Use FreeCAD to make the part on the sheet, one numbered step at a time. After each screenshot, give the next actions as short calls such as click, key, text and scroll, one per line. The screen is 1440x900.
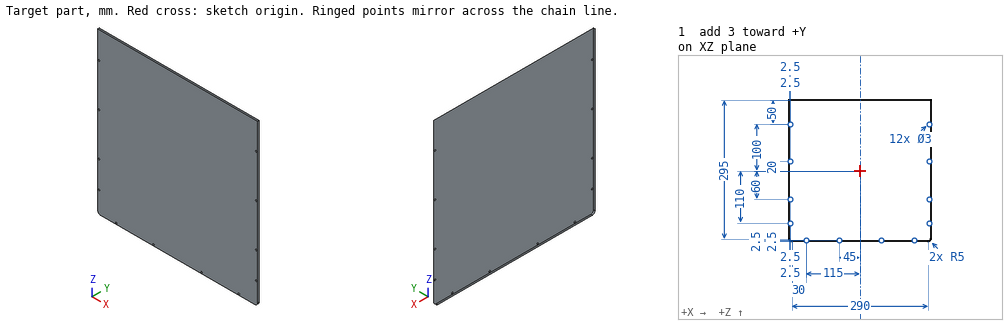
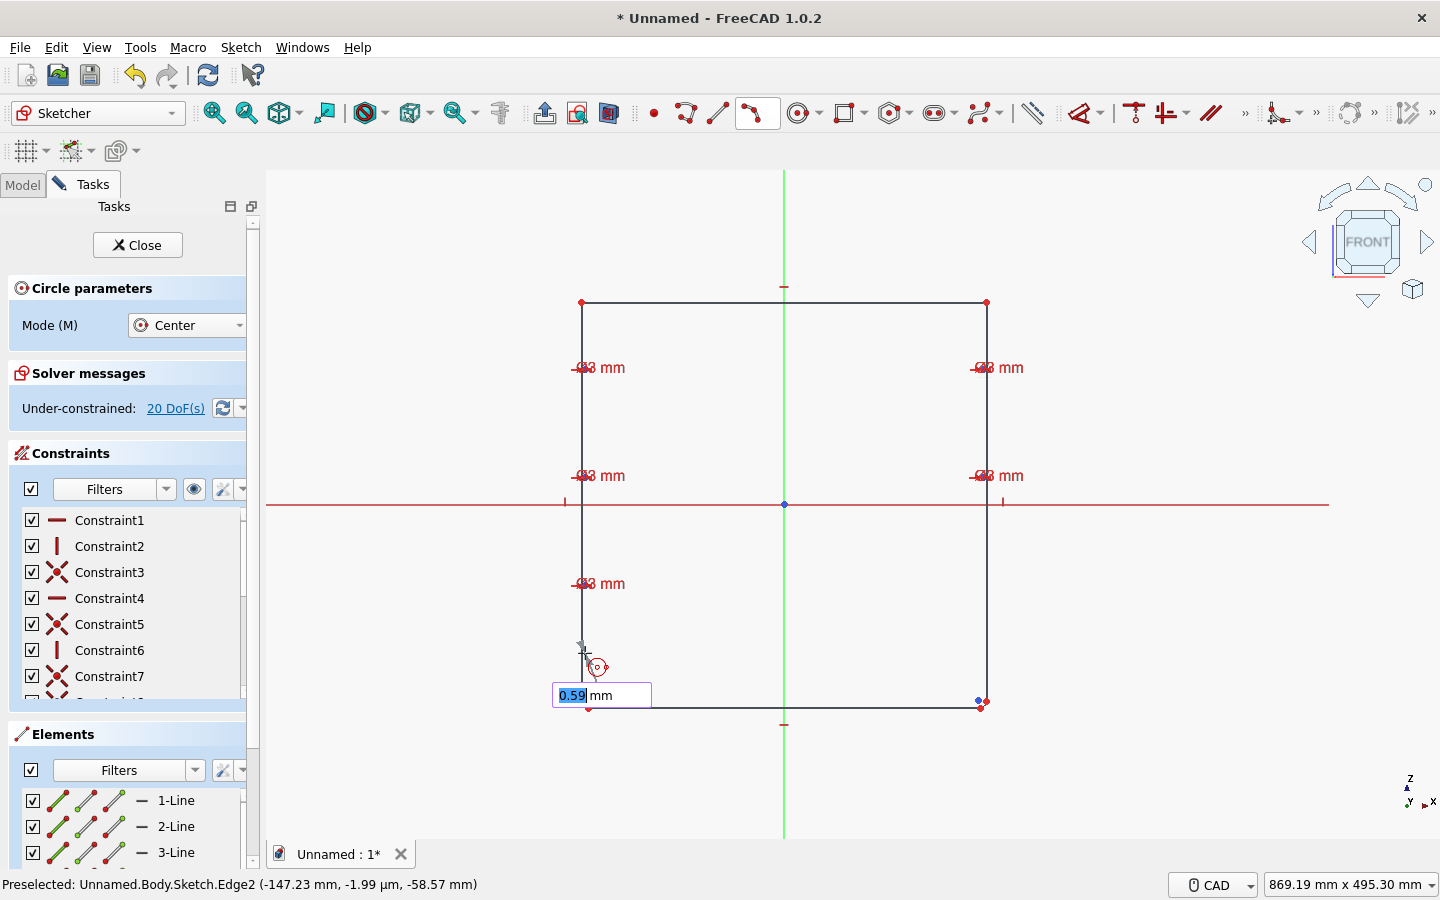
scroll(587, 652, up, 6)
move(585, 650)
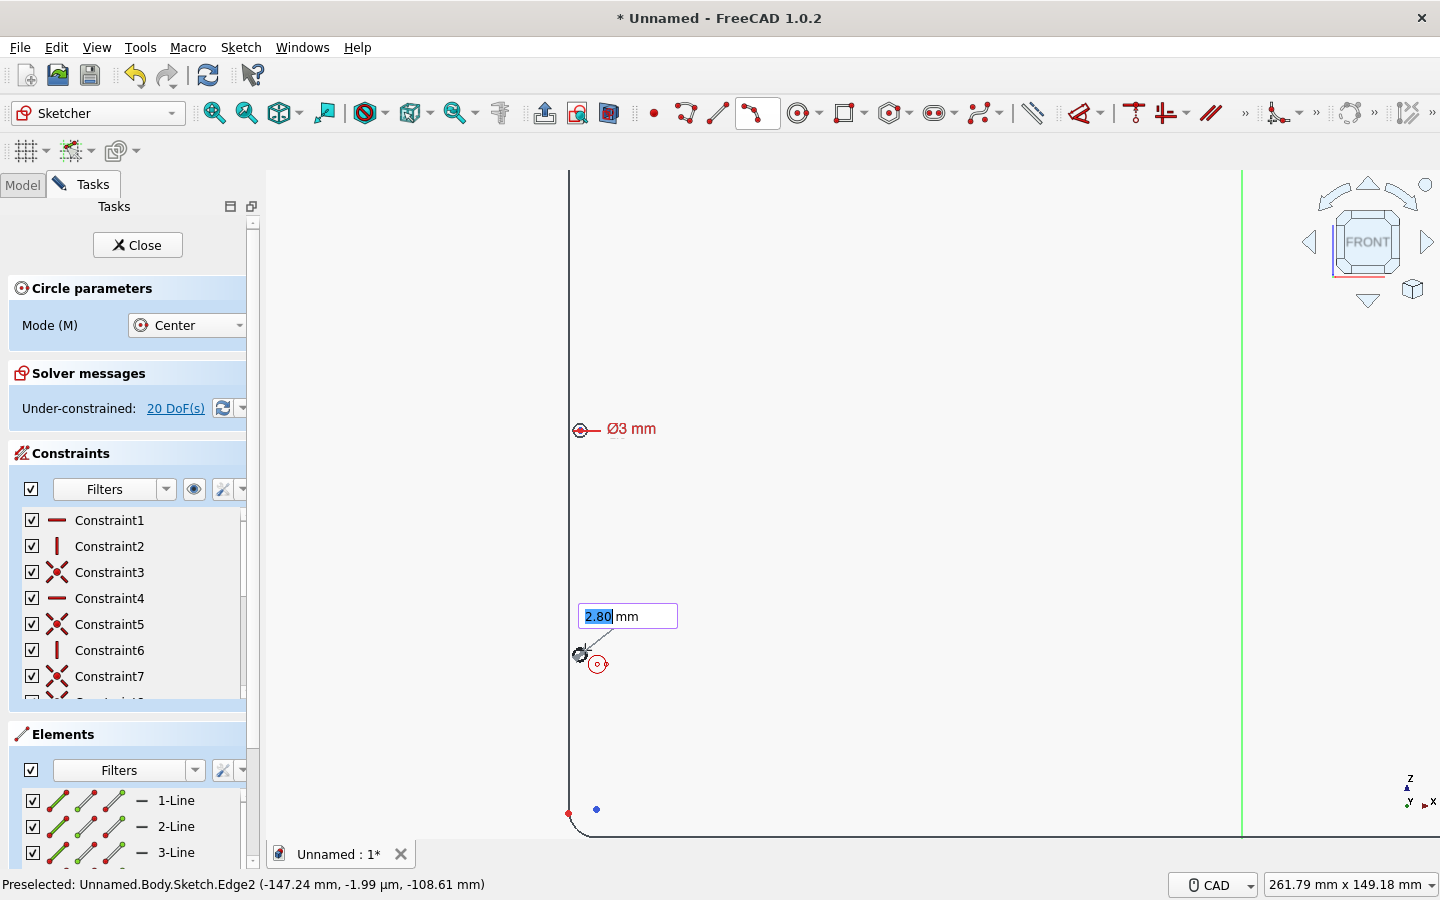
text(3)
key(Return)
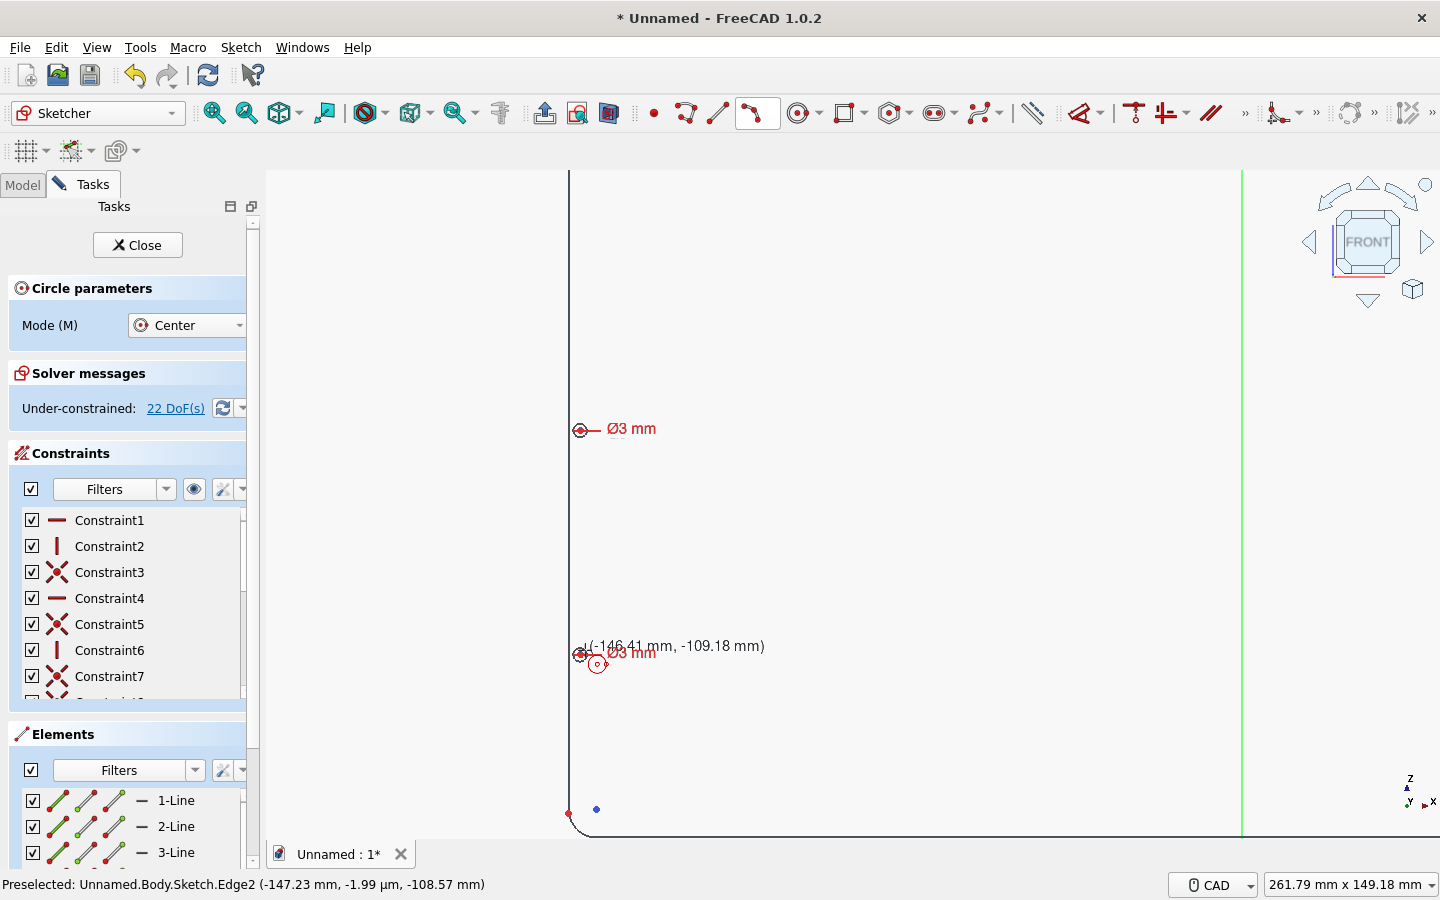
scroll(587, 652, down, 6)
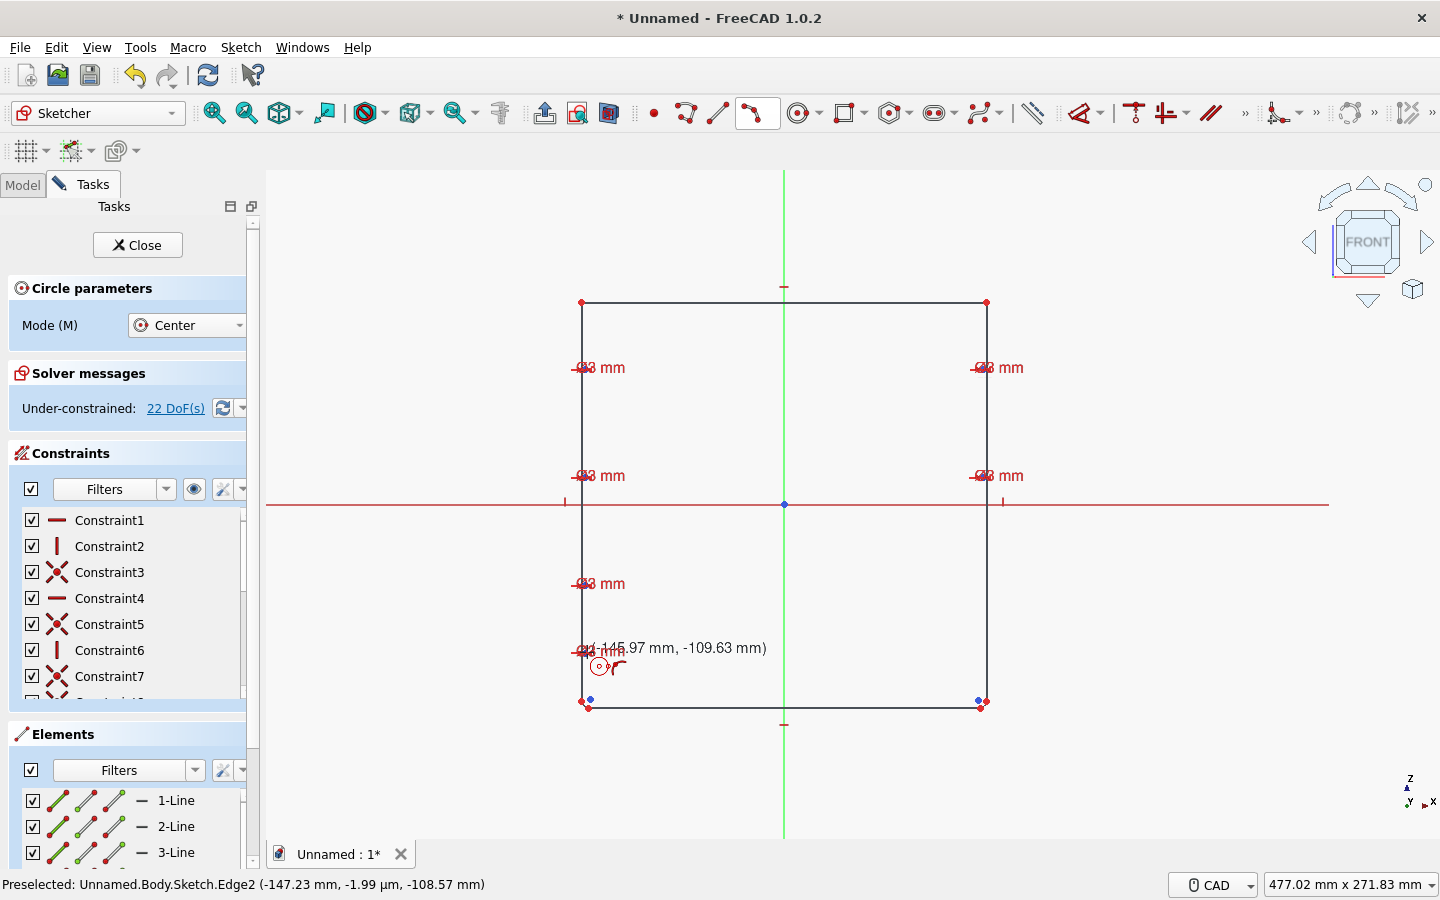
scroll(629, 704, up, 13)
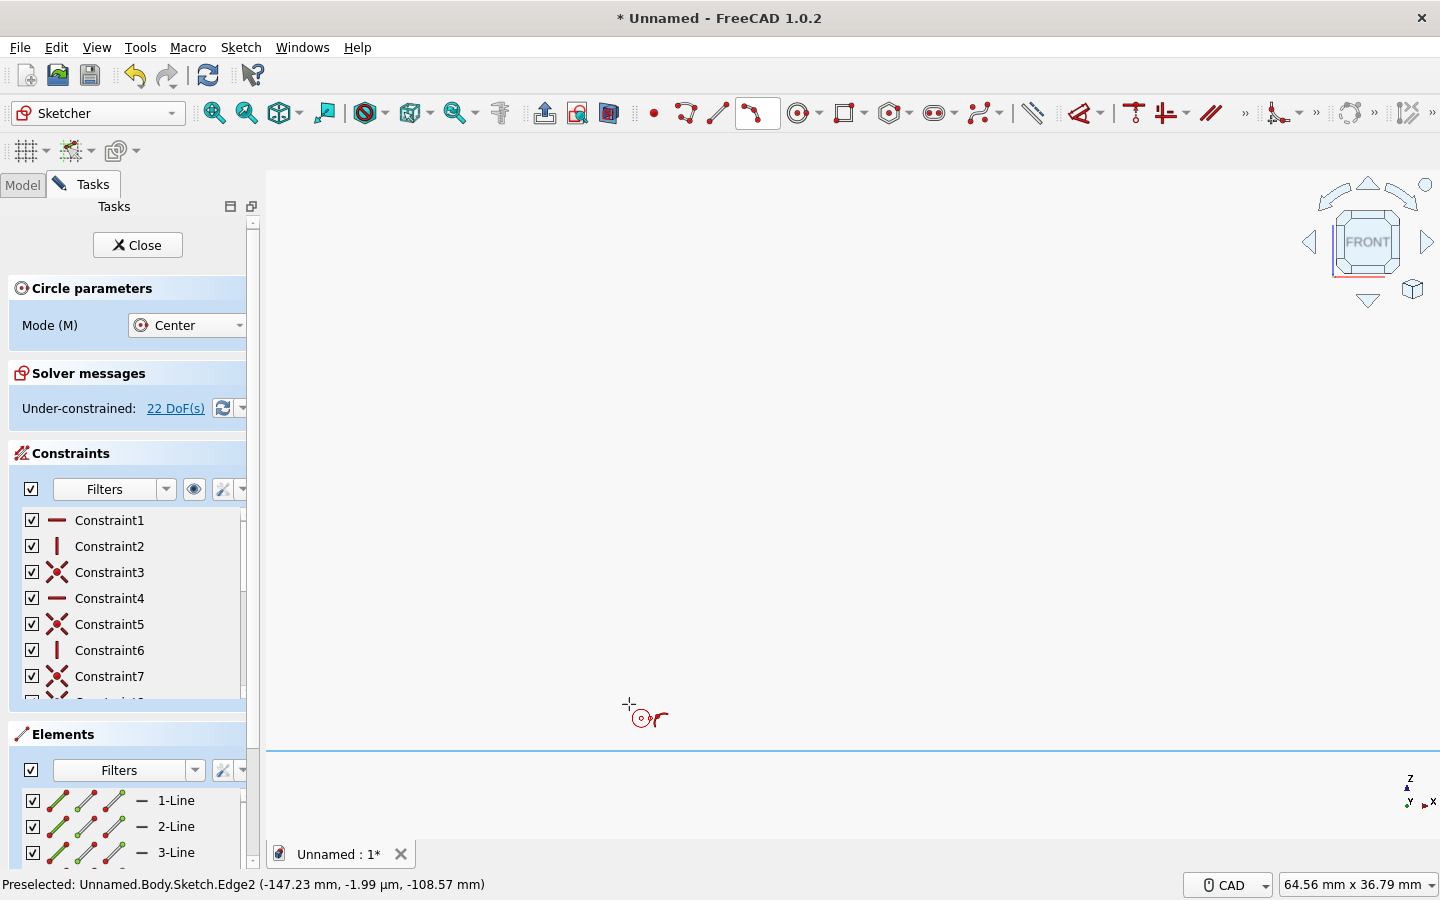
click(625, 694)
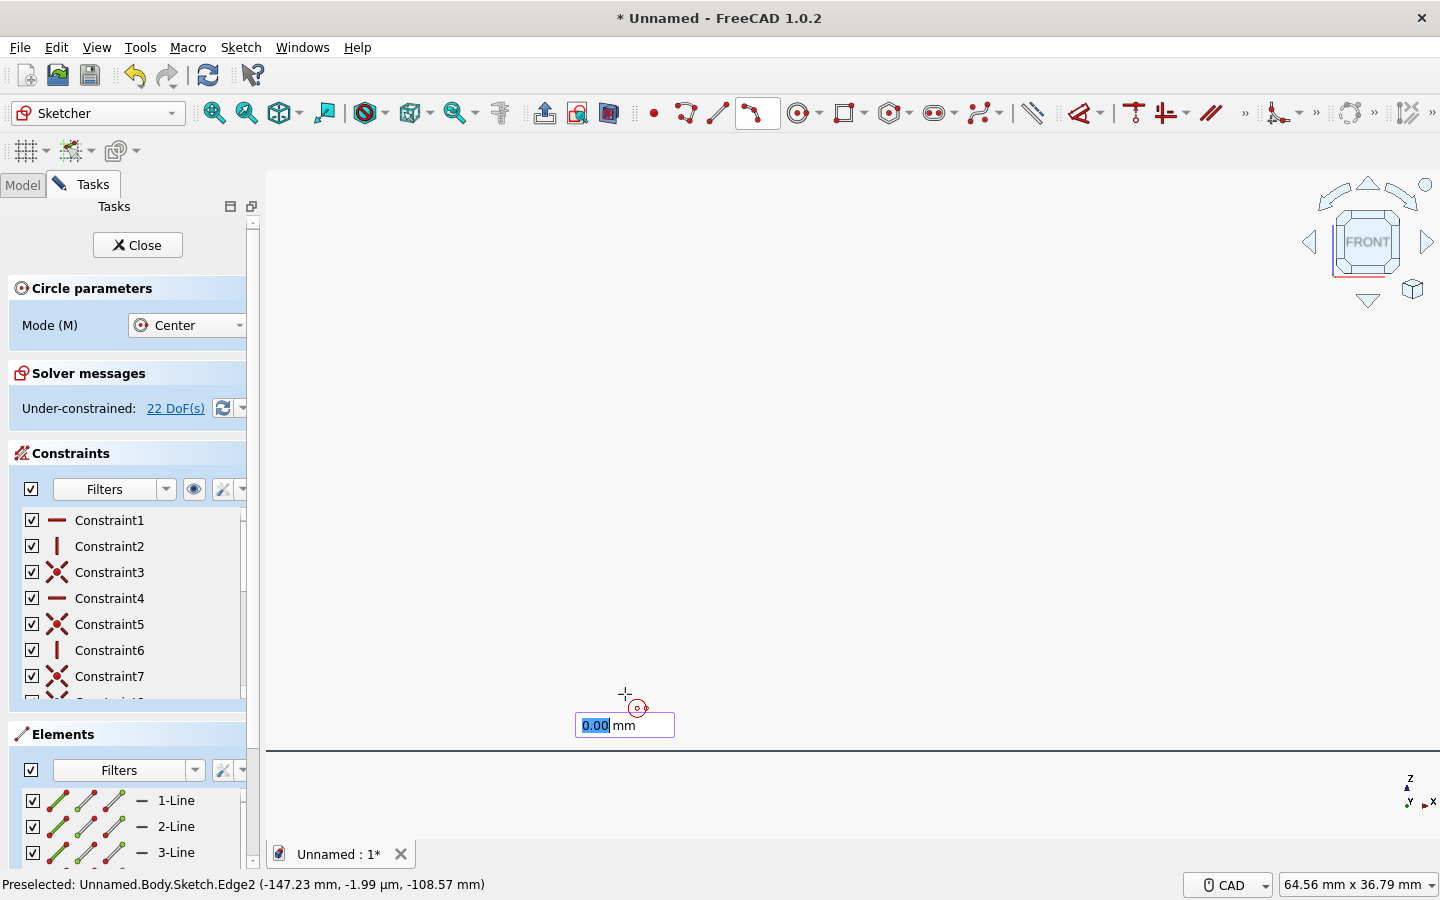
scroll(629, 705, down, 13)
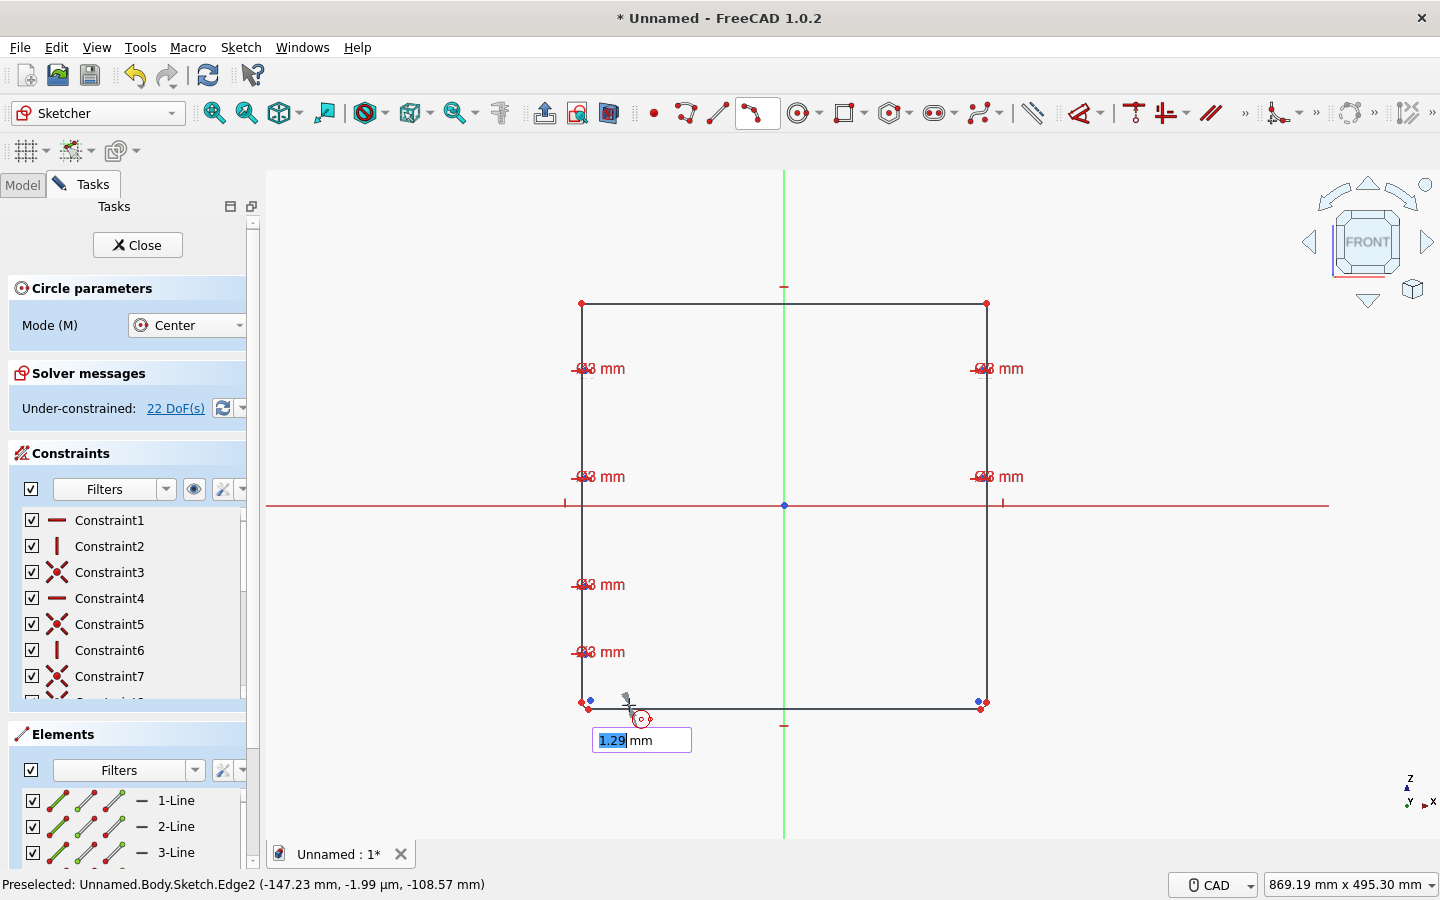
scroll(630, 703, up, 6)
move(631, 703)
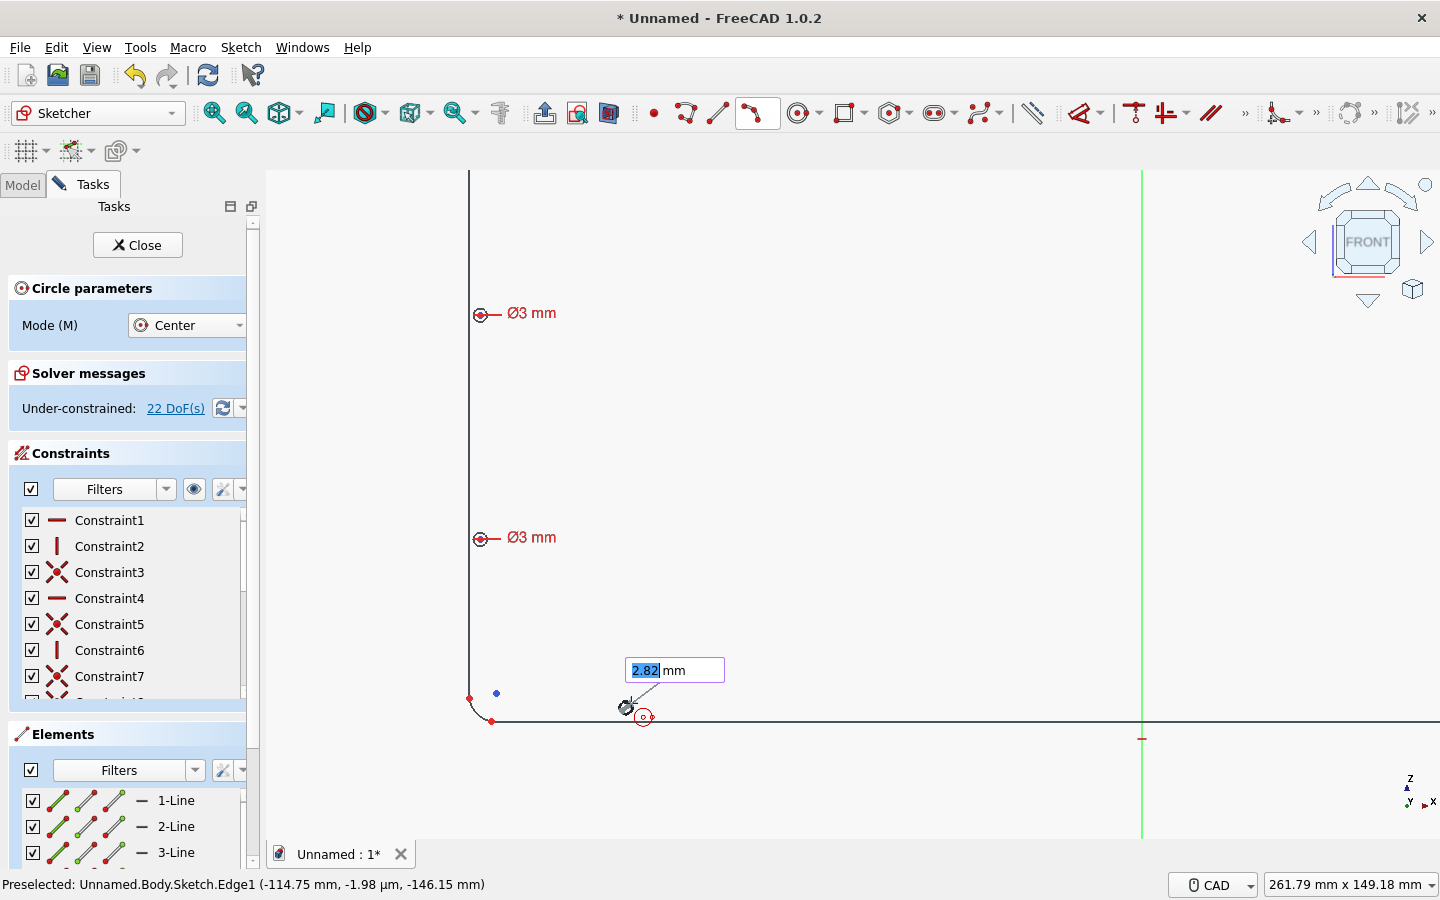
text(3)
key(Return)